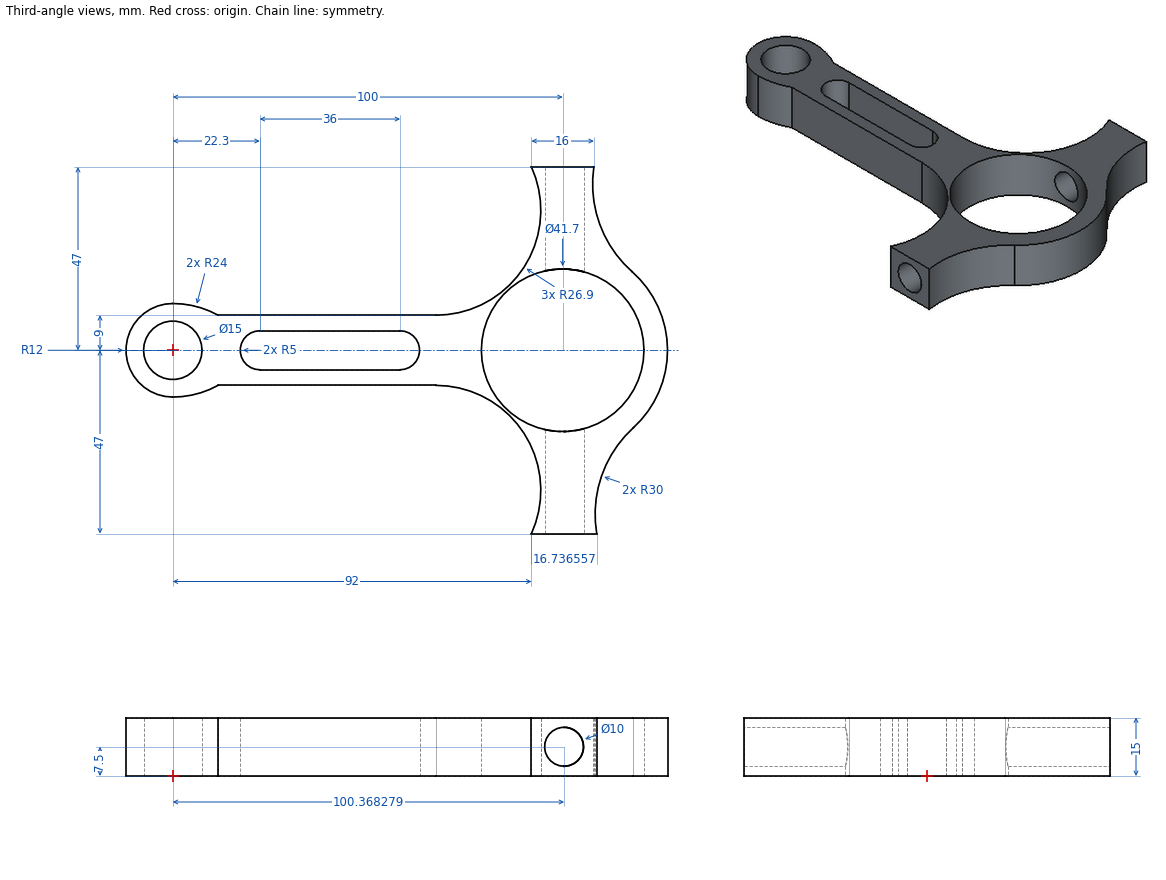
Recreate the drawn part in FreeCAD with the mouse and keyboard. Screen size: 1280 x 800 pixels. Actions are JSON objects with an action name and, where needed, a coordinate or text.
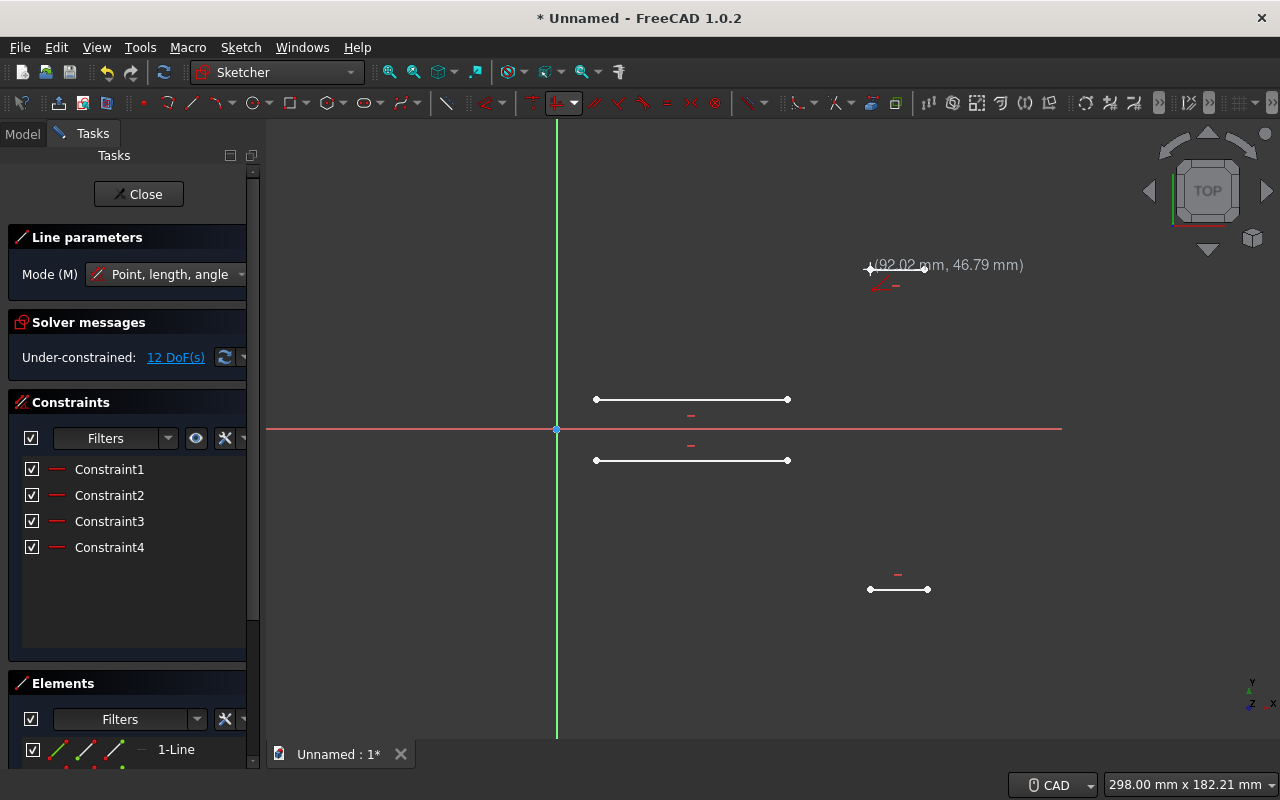
{"action": "left_click", "coordinate": [216, 104]}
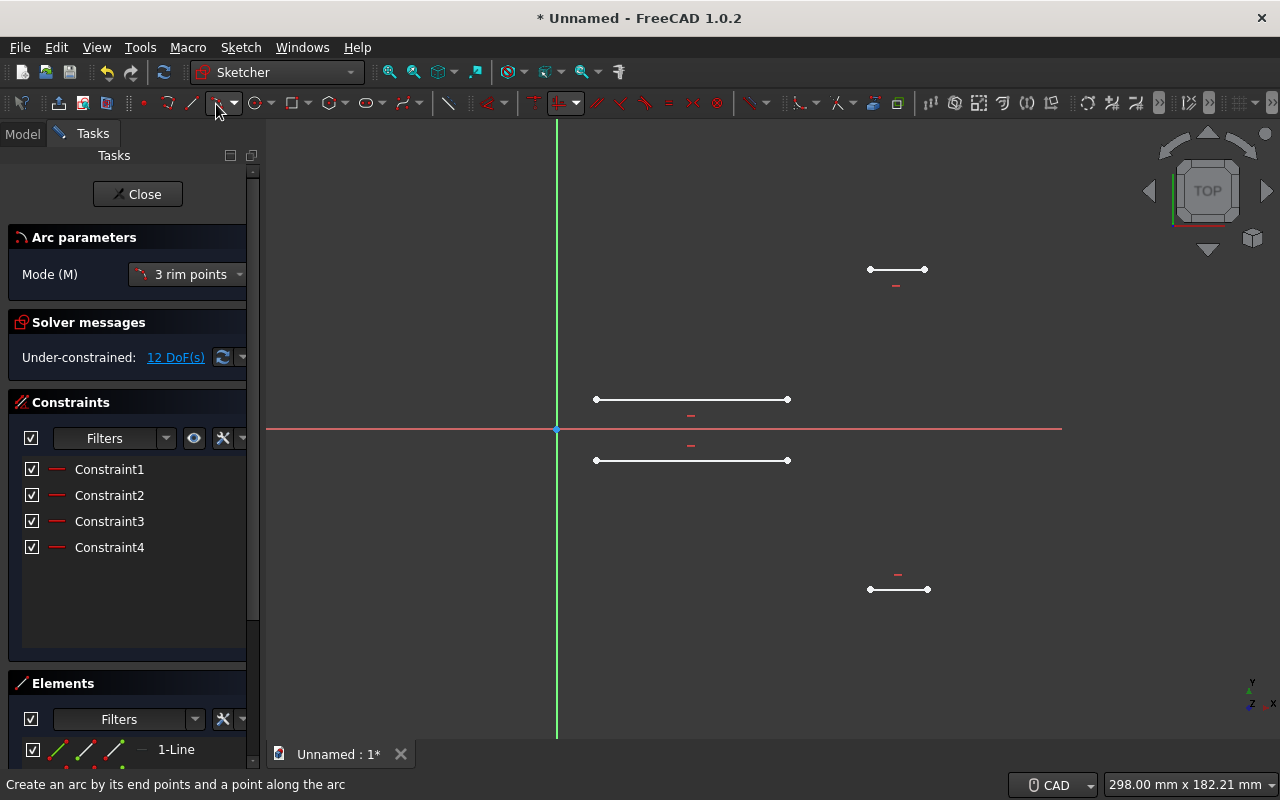
{"action": "left_click", "coordinate": [596, 400]}
{"action": "left_click", "coordinate": [557, 388]}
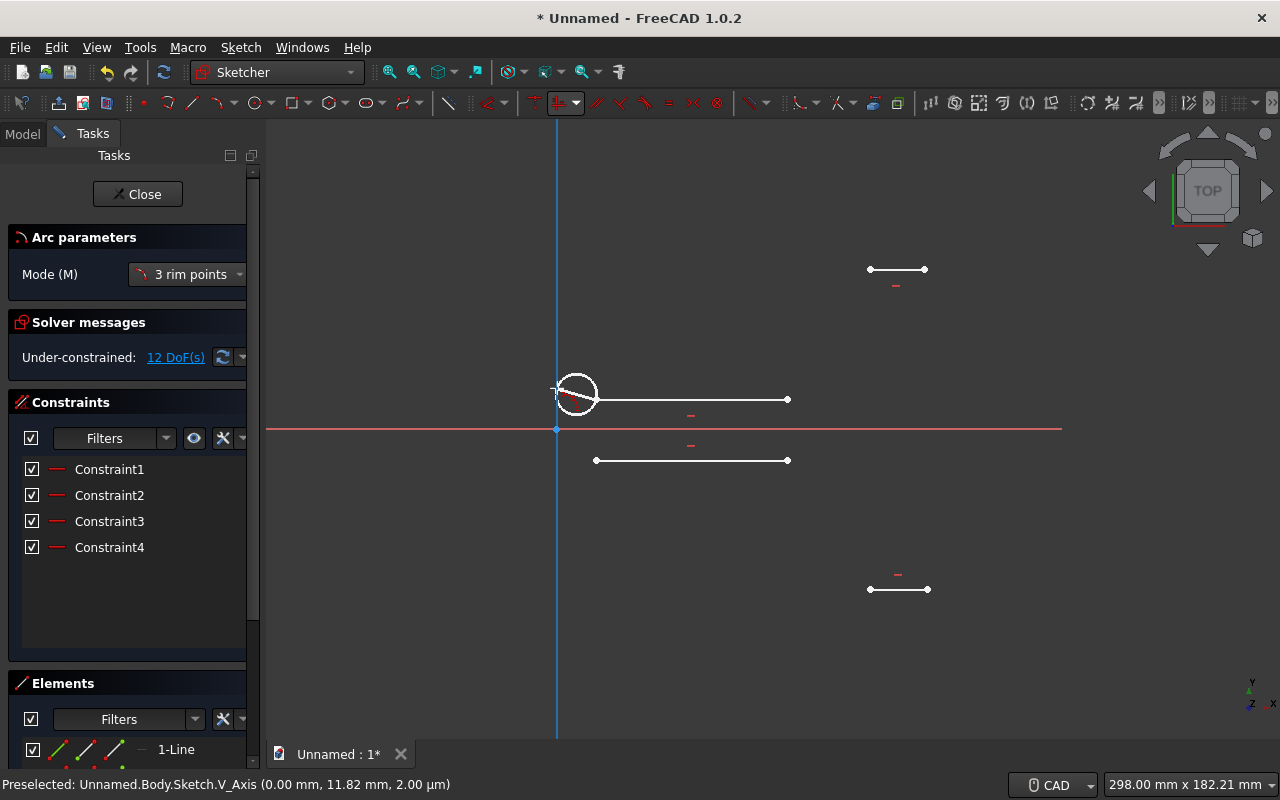
{"action": "scroll", "coordinate": [577, 391], "scroll_direction": "up", "scroll_amount": 10}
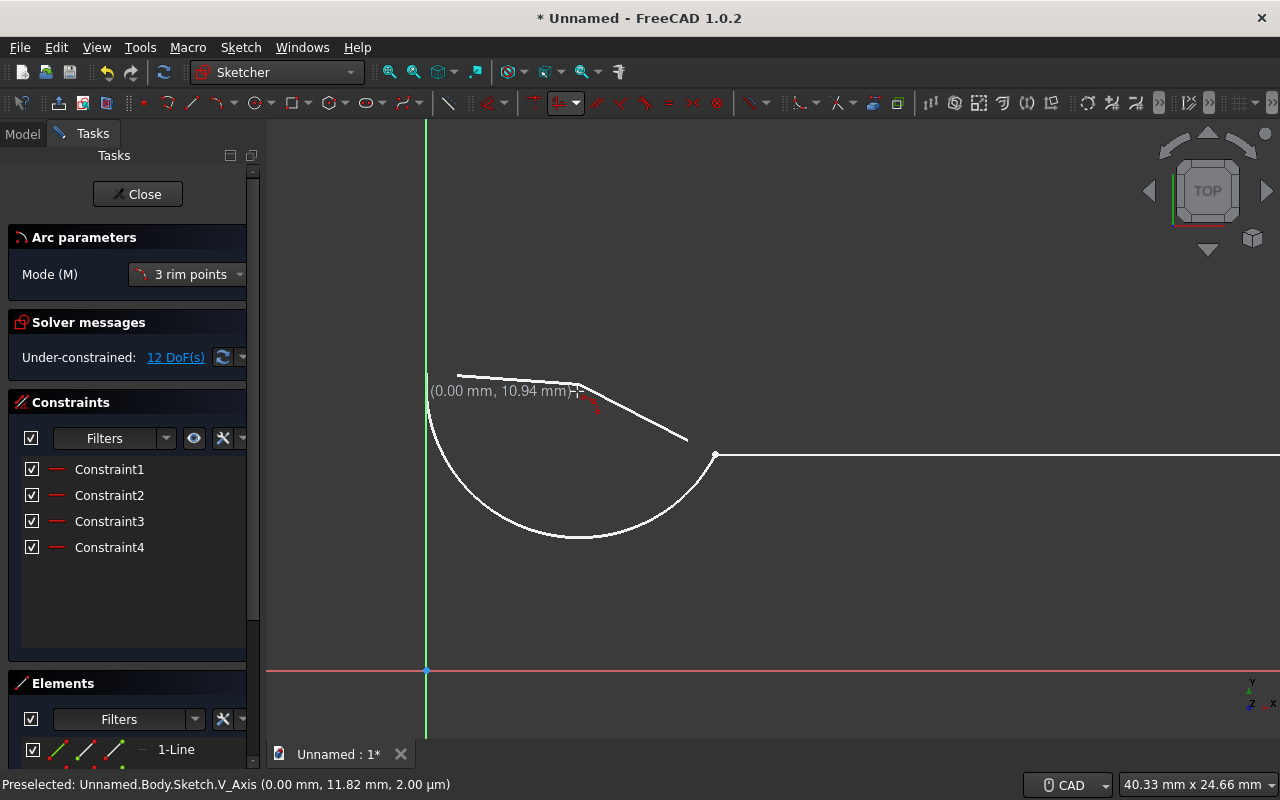
{"action": "left_click", "coordinate": [577, 388]}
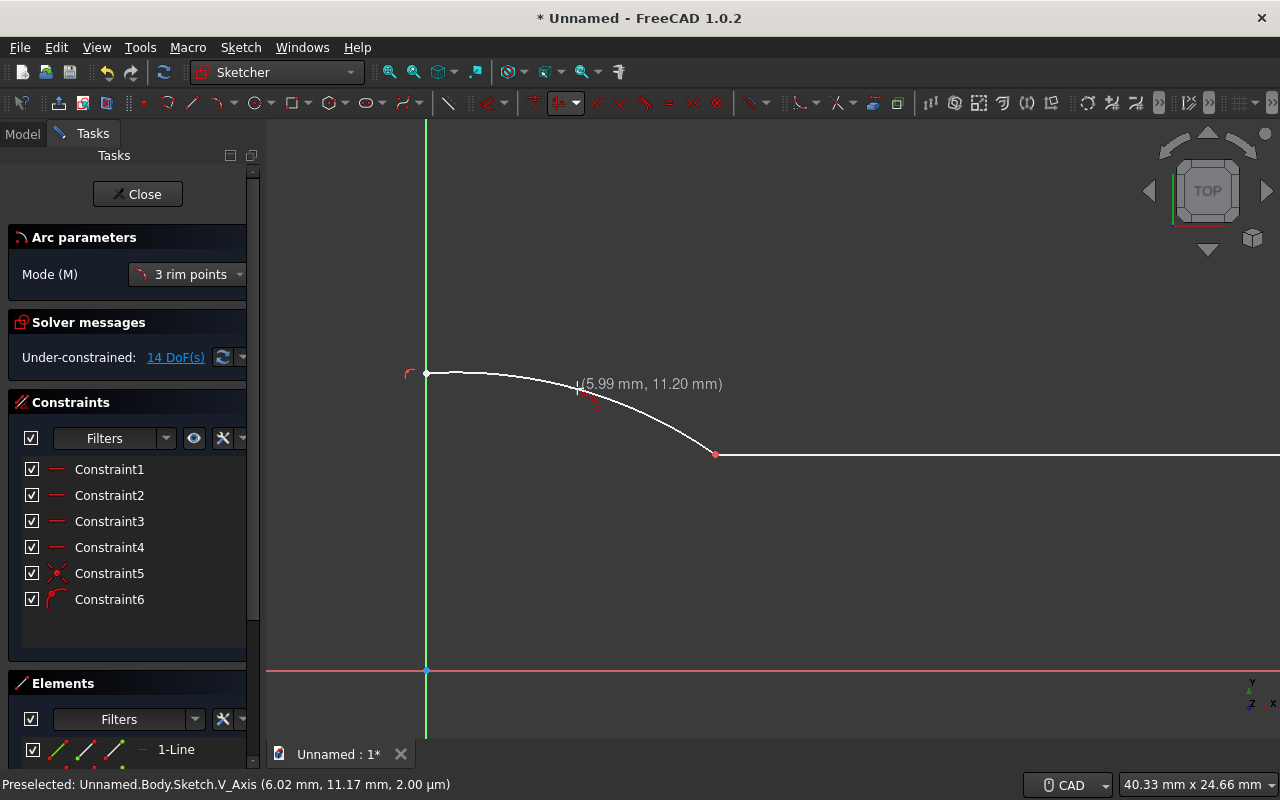
{"action": "scroll", "coordinate": [474, 381], "scroll_direction": "down", "scroll_amount": 9}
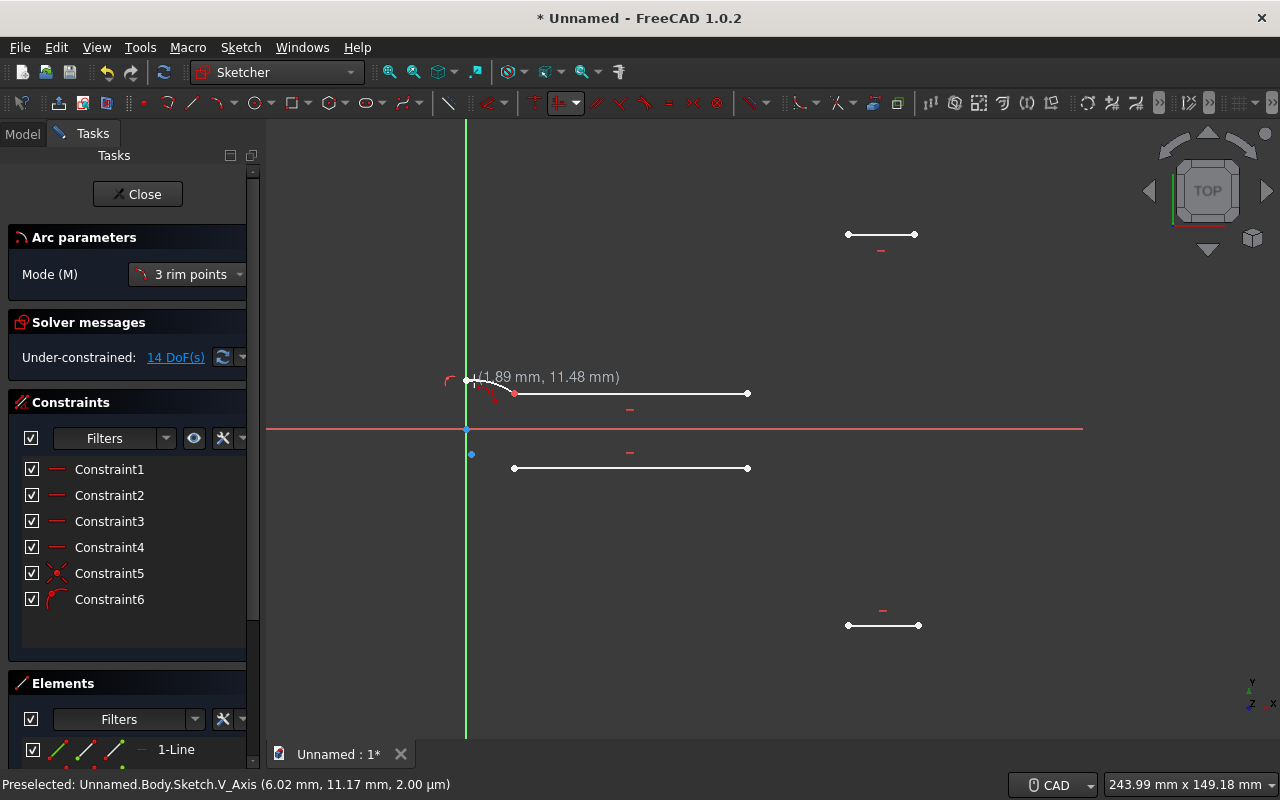
{"action": "left_click", "coordinate": [466, 380]}
{"action": "left_click", "coordinate": [466, 479]}
{"action": "left_click", "coordinate": [426, 400]}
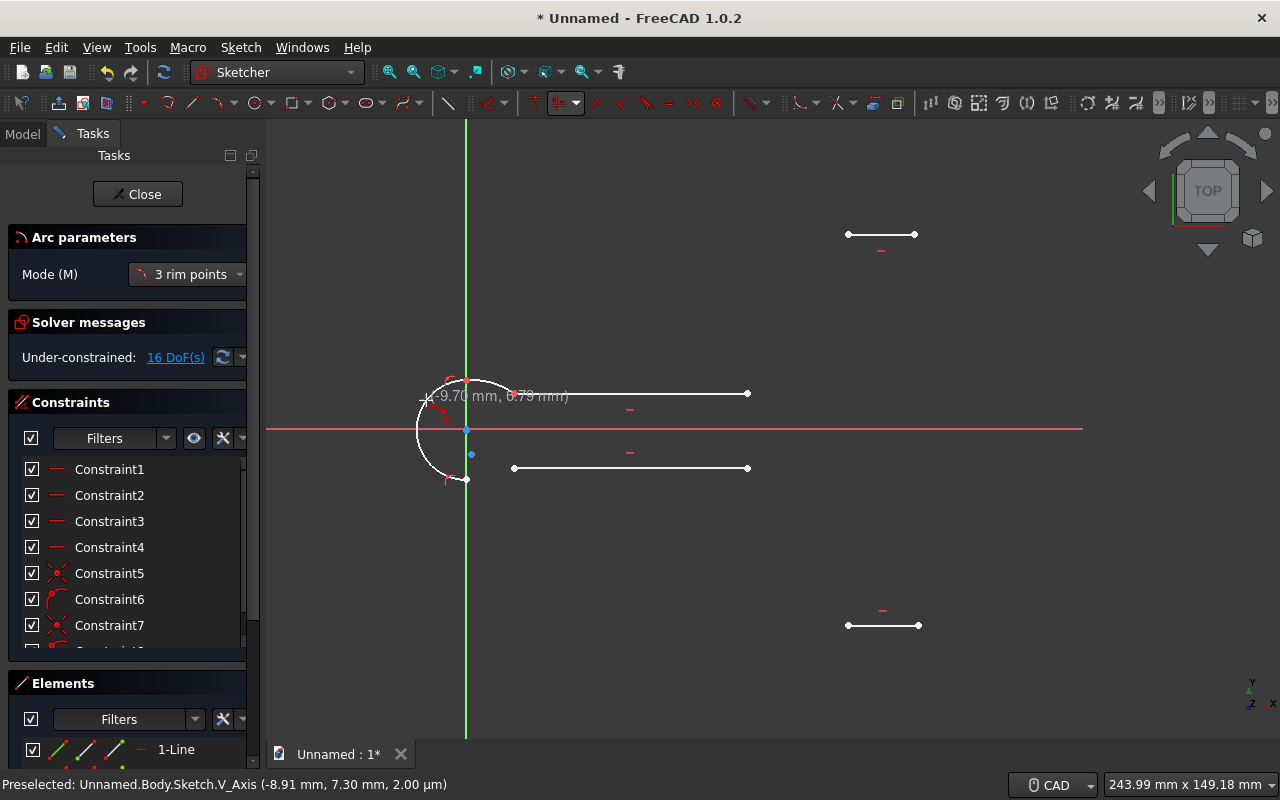
{"action": "left_click", "coordinate": [466, 480]}
{"action": "left_click", "coordinate": [514, 468]}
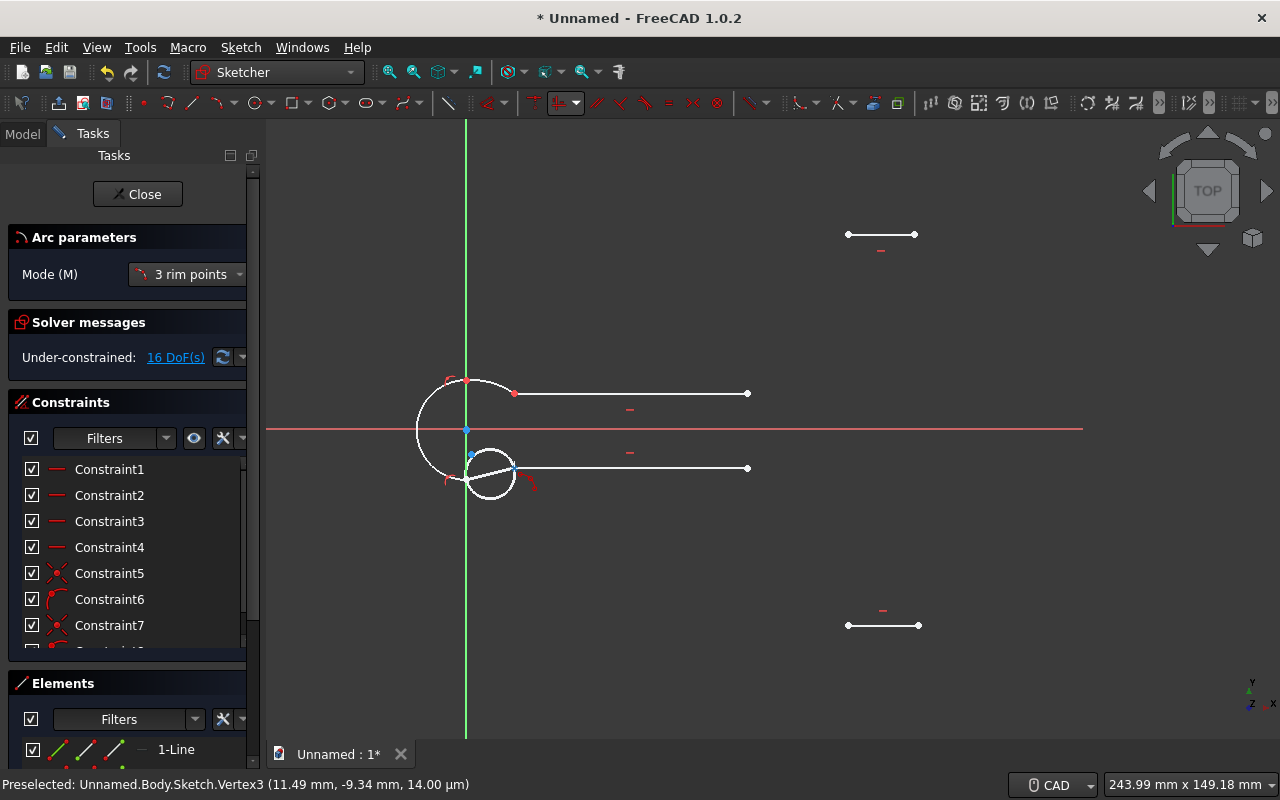
{"action": "scroll", "coordinate": [491, 476], "scroll_direction": "up", "scroll_amount": 9}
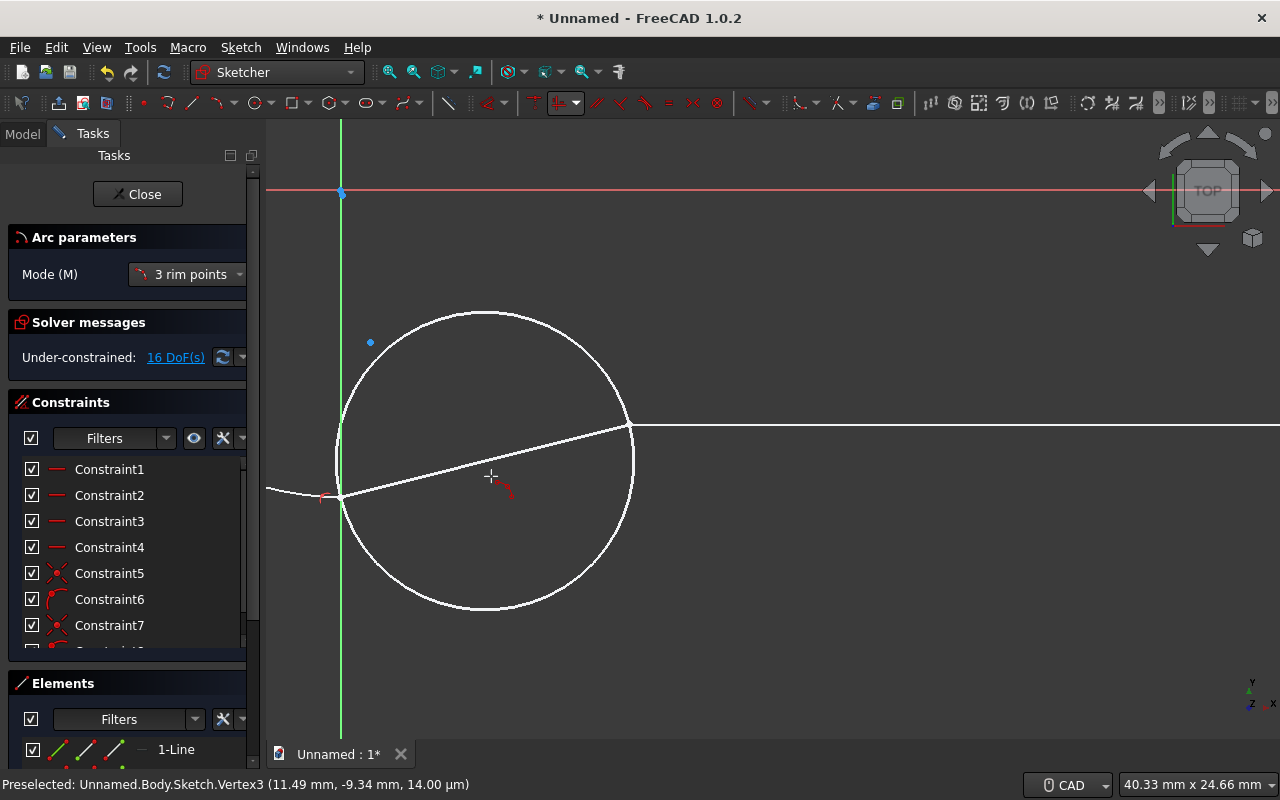
{"action": "left_click", "coordinate": [491, 473]}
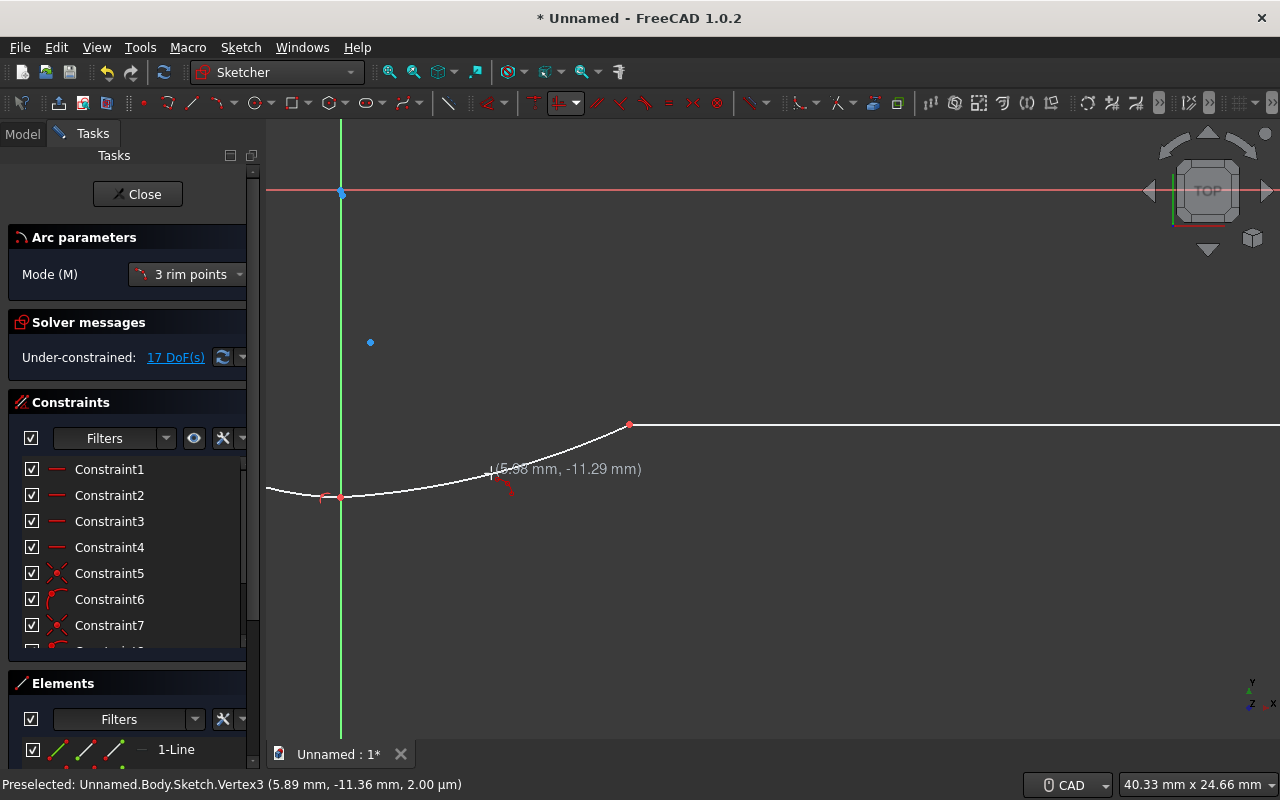
{"action": "scroll", "coordinate": [491, 476], "scroll_direction": "down", "scroll_amount": 9}